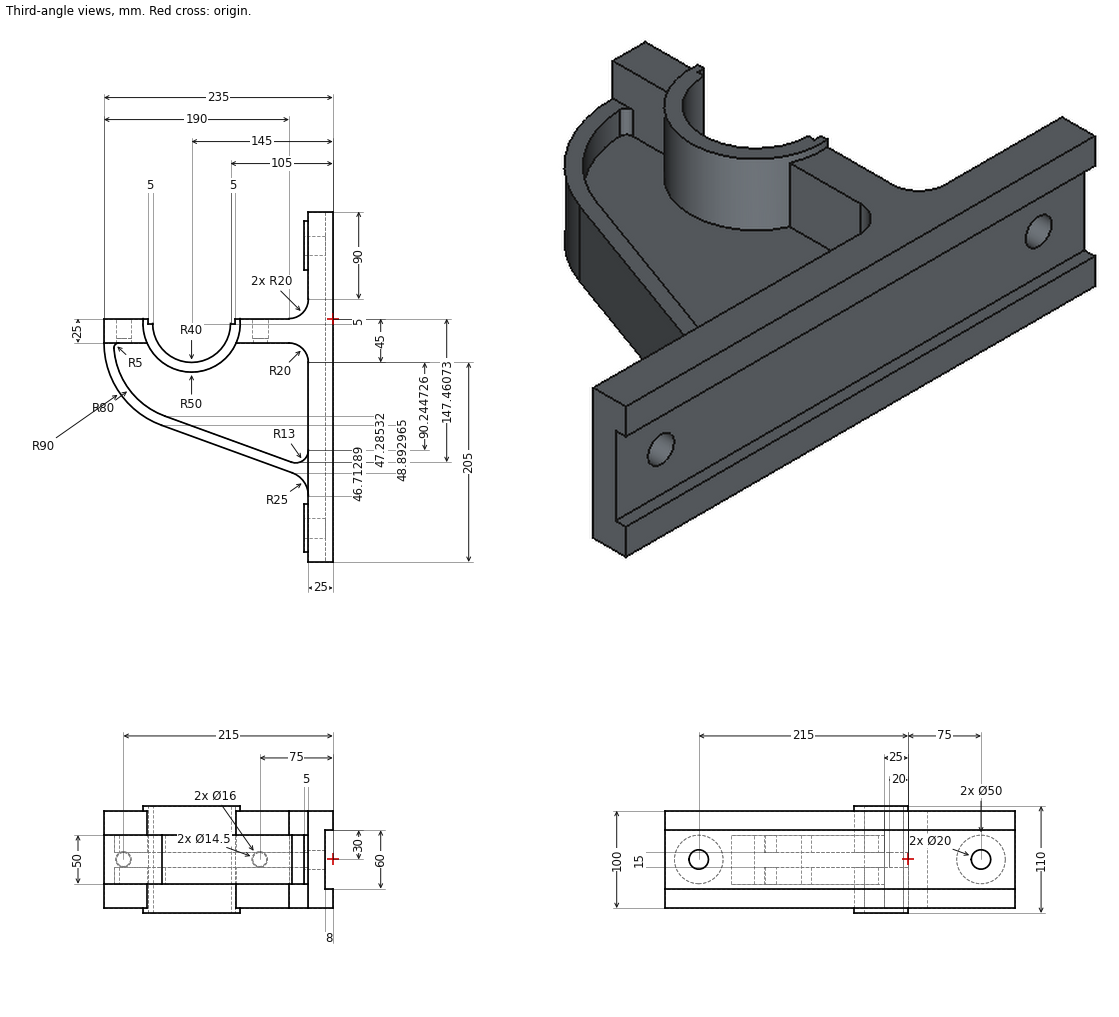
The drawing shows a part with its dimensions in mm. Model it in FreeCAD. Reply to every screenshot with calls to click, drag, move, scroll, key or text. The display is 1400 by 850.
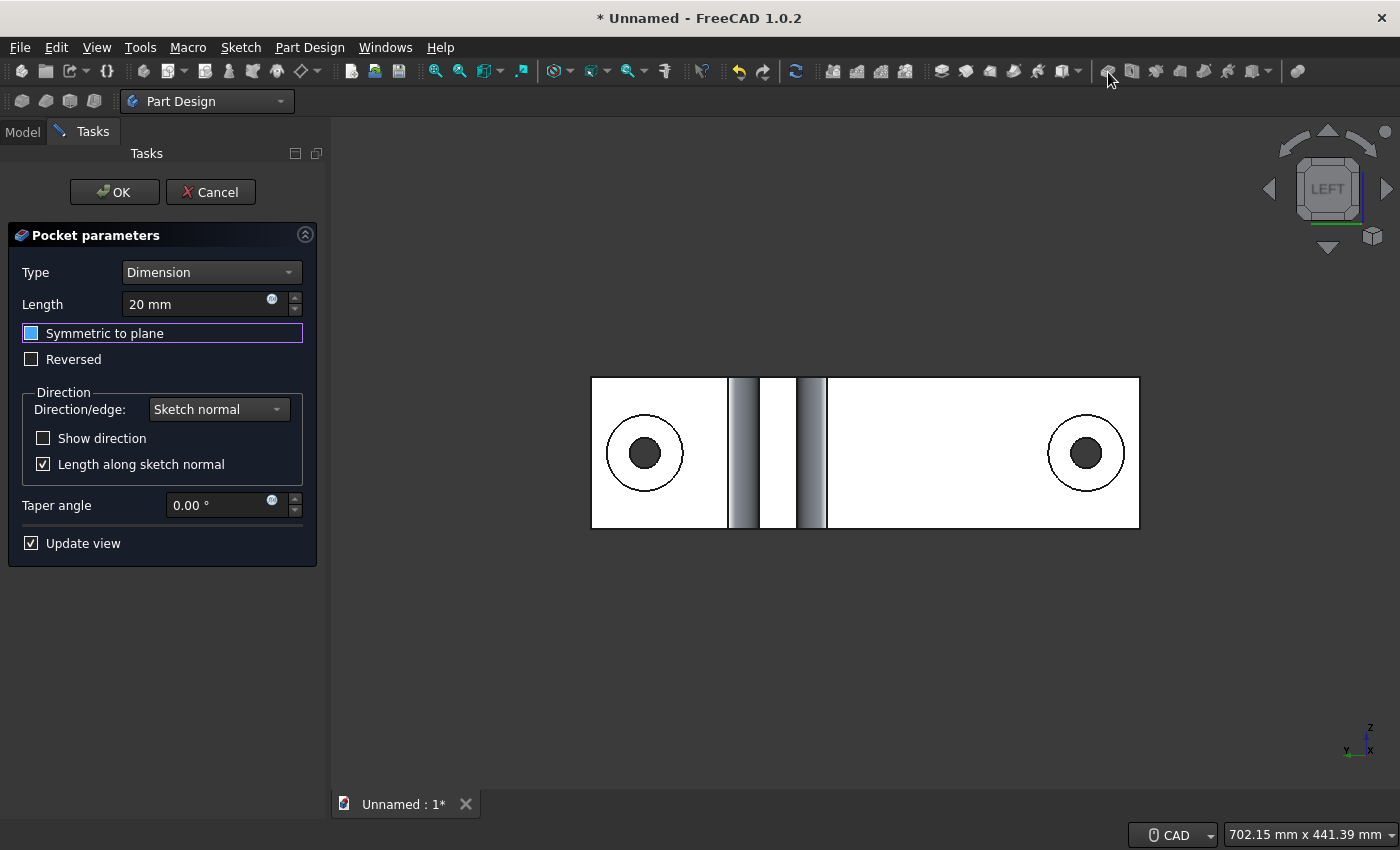
click(30, 359)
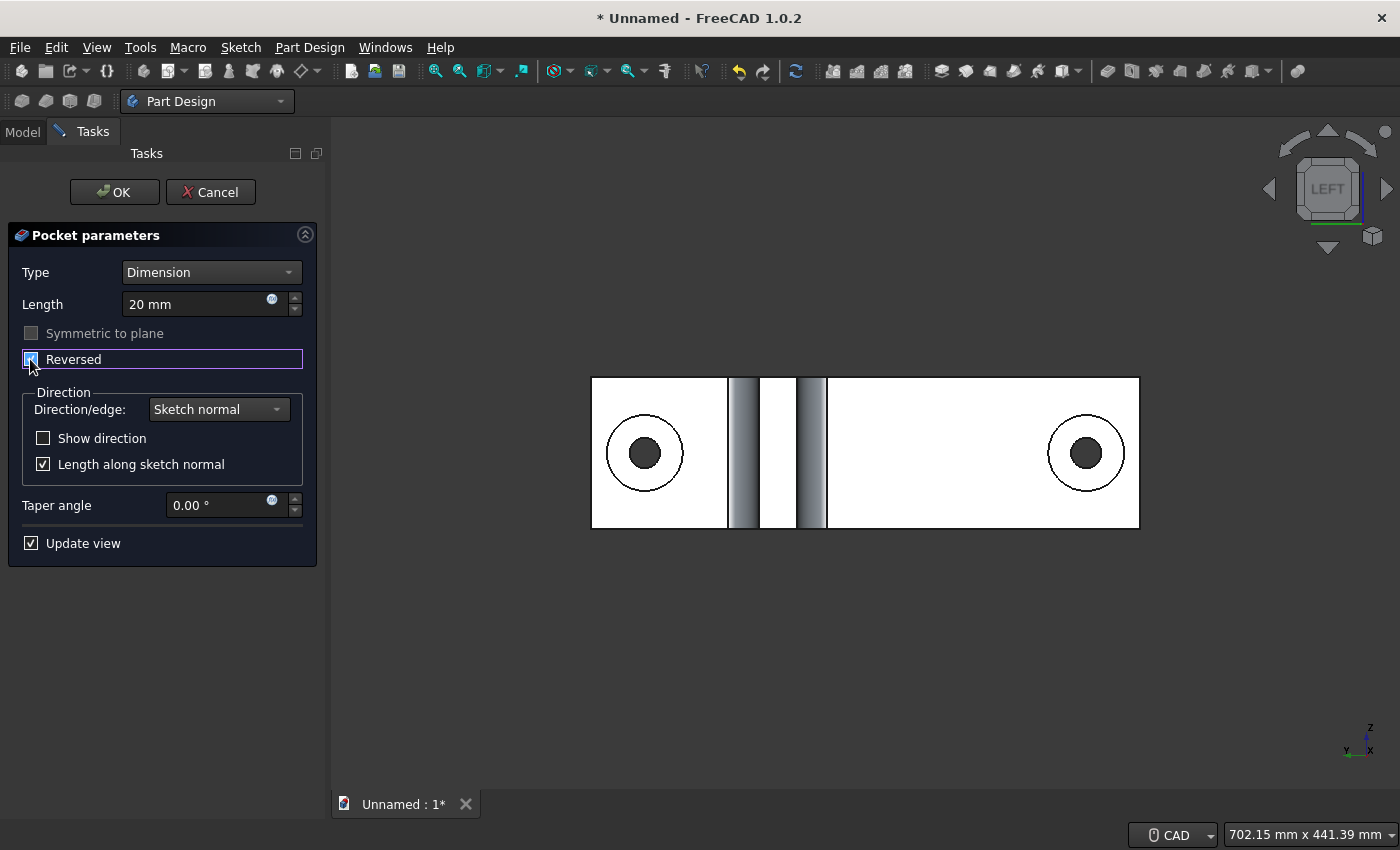
click(115, 192)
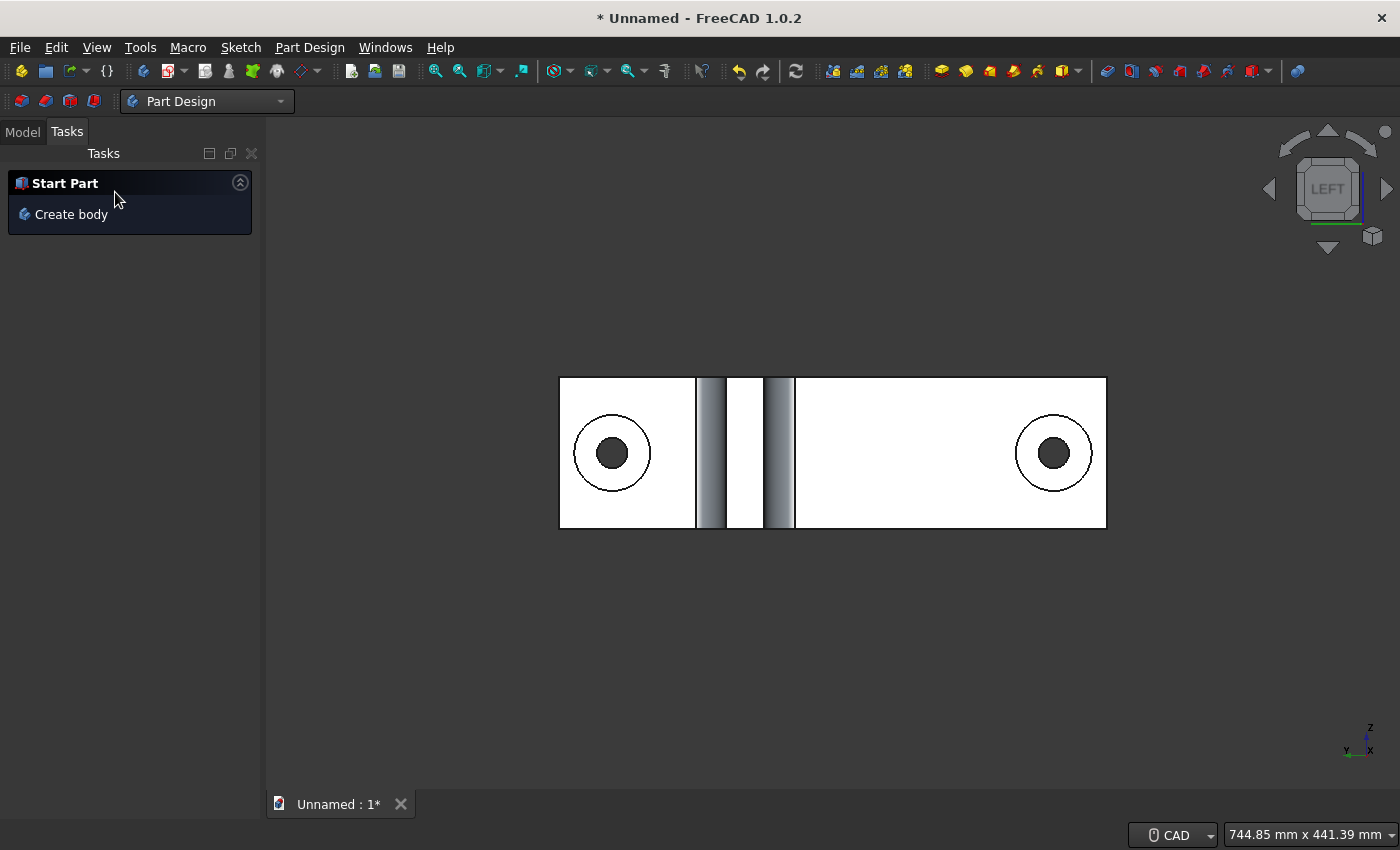
click(168, 72)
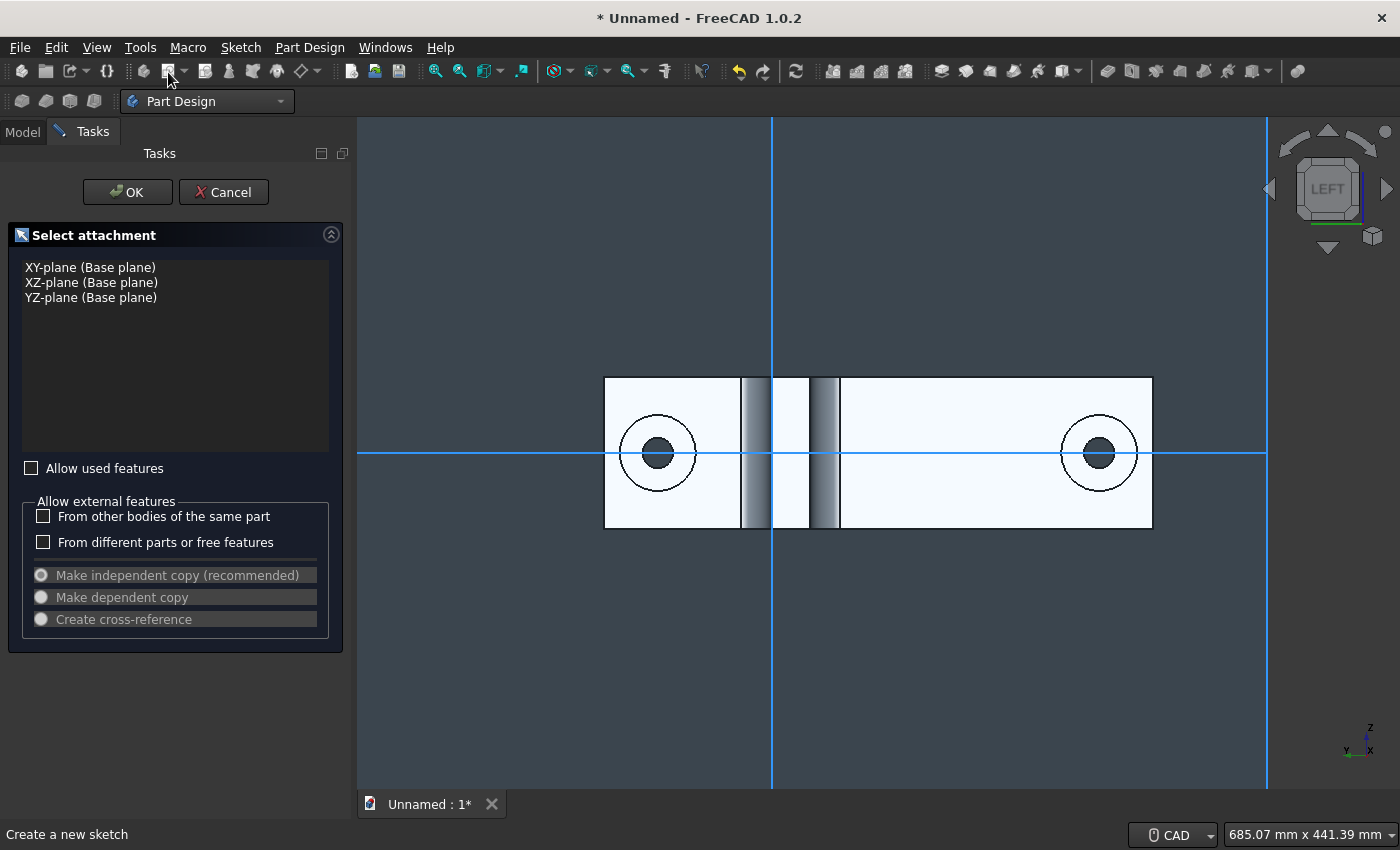
click(82, 268)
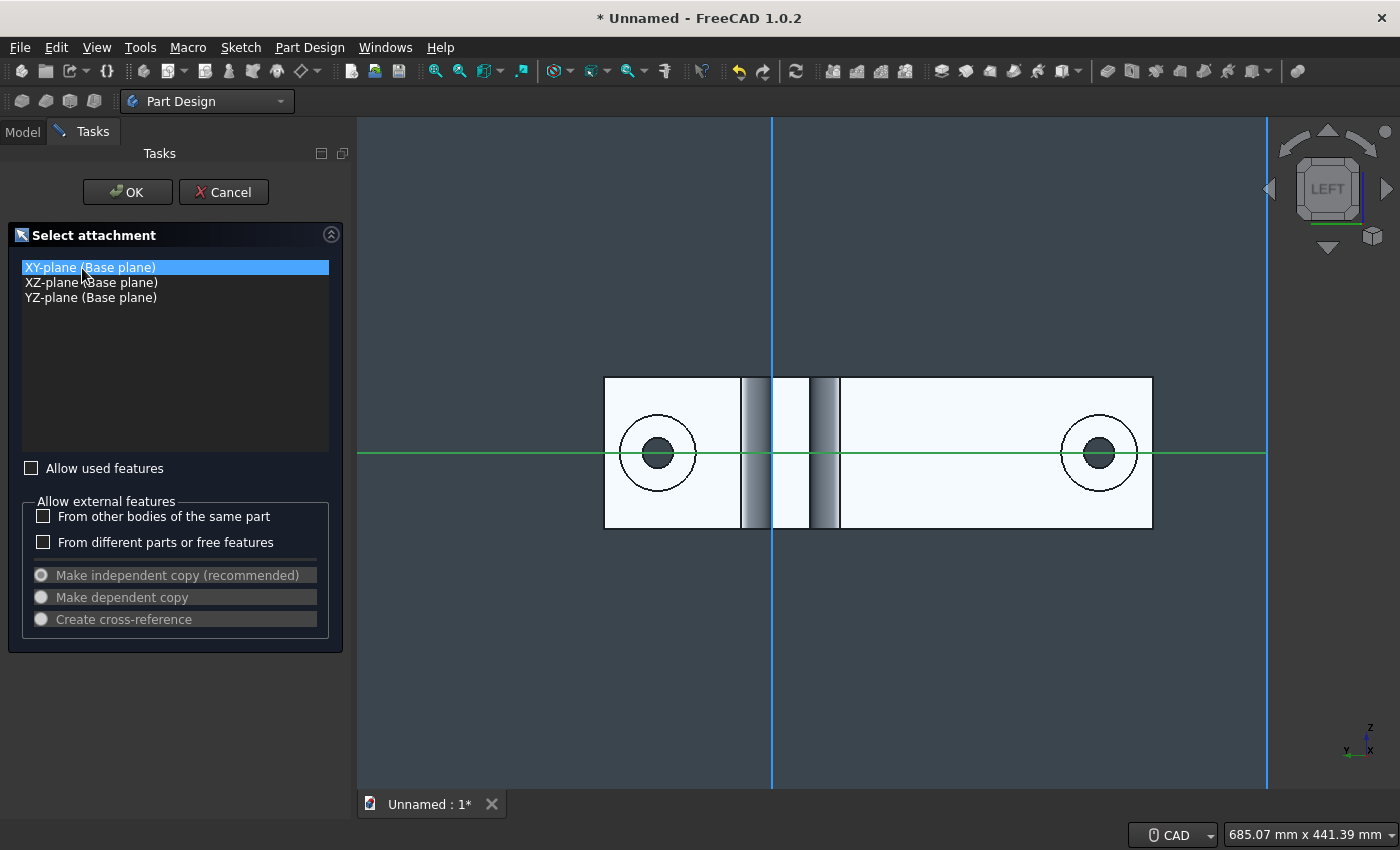
click(128, 192)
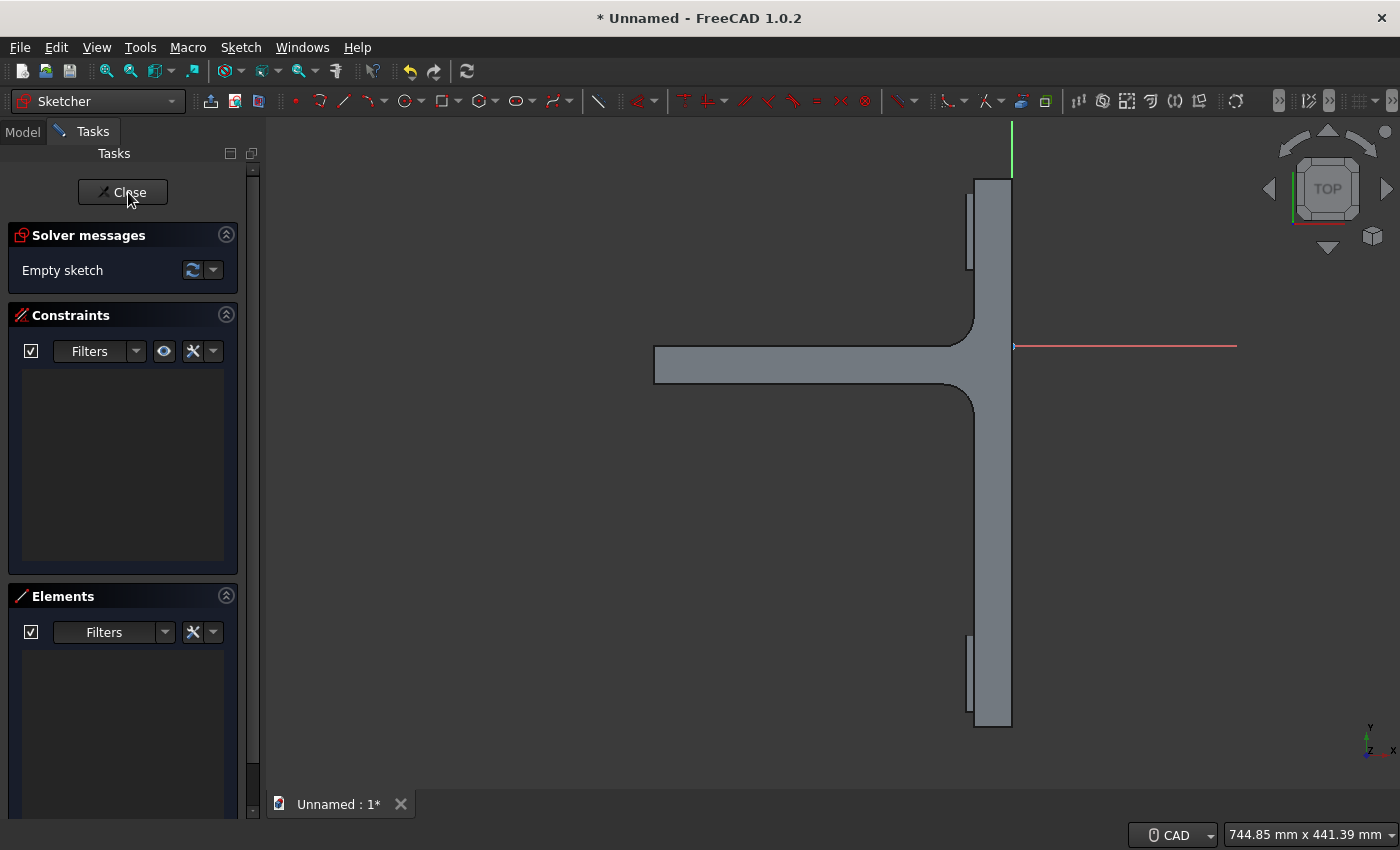
click(260, 102)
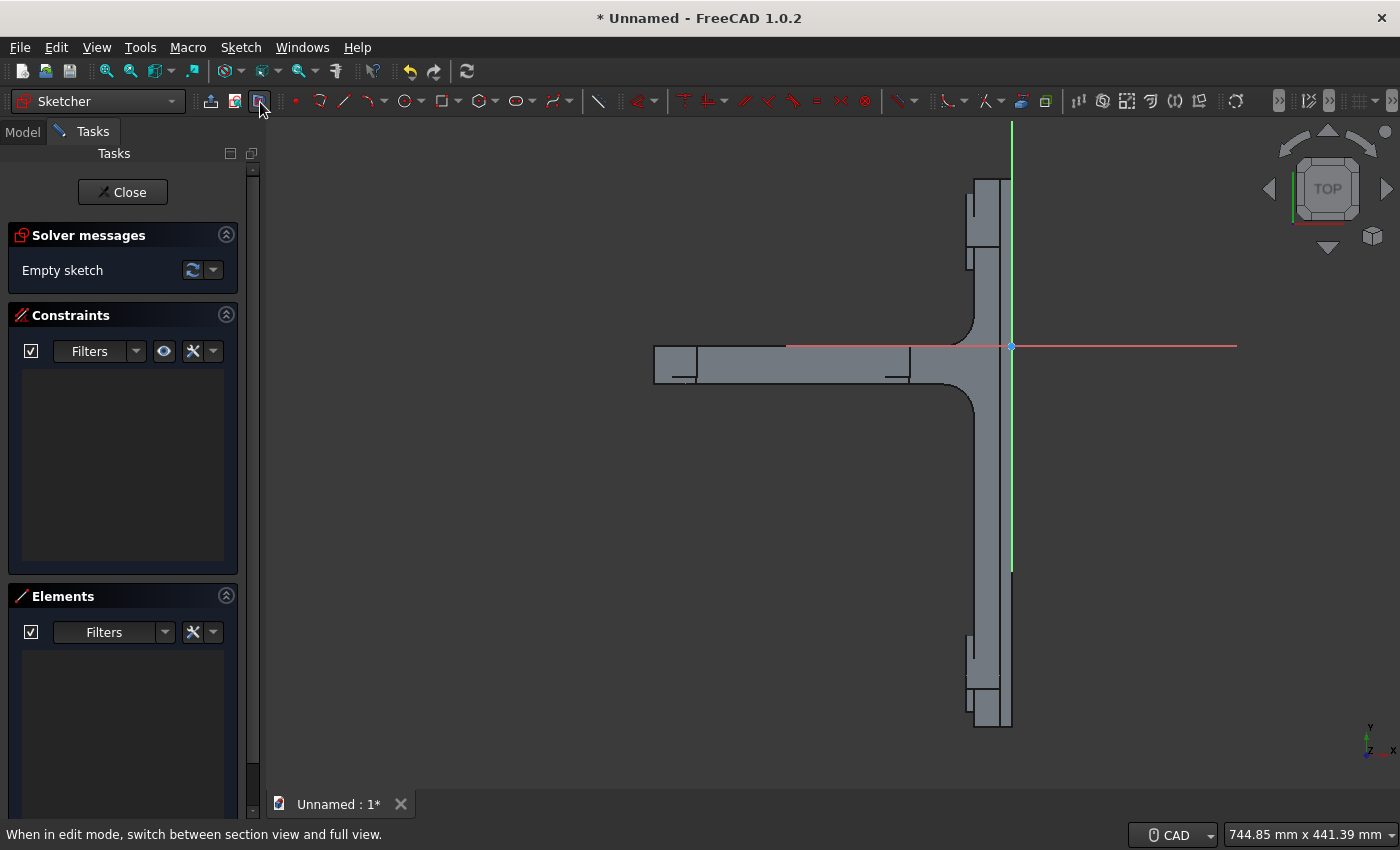
scroll(945, 335, up, 4)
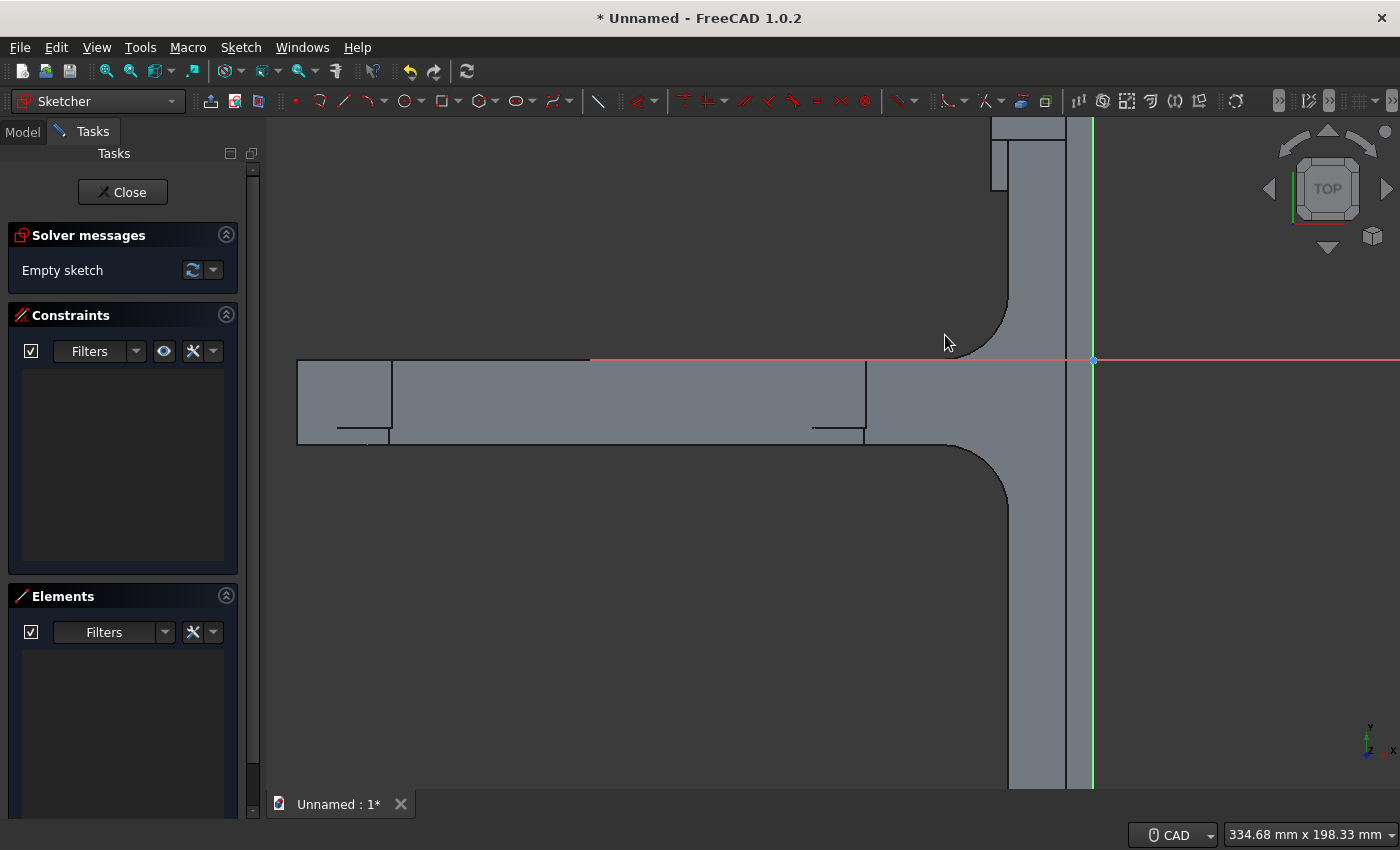
click(344, 102)